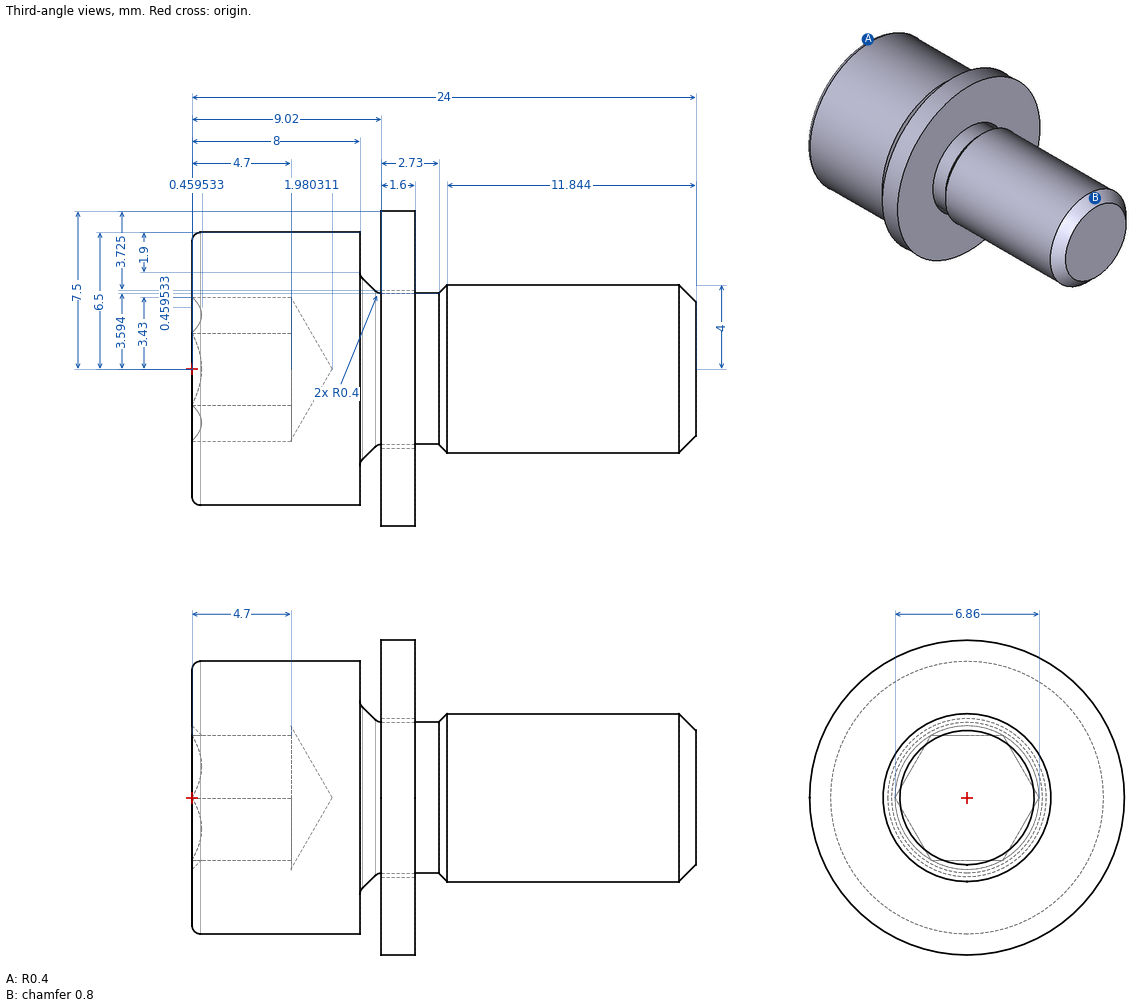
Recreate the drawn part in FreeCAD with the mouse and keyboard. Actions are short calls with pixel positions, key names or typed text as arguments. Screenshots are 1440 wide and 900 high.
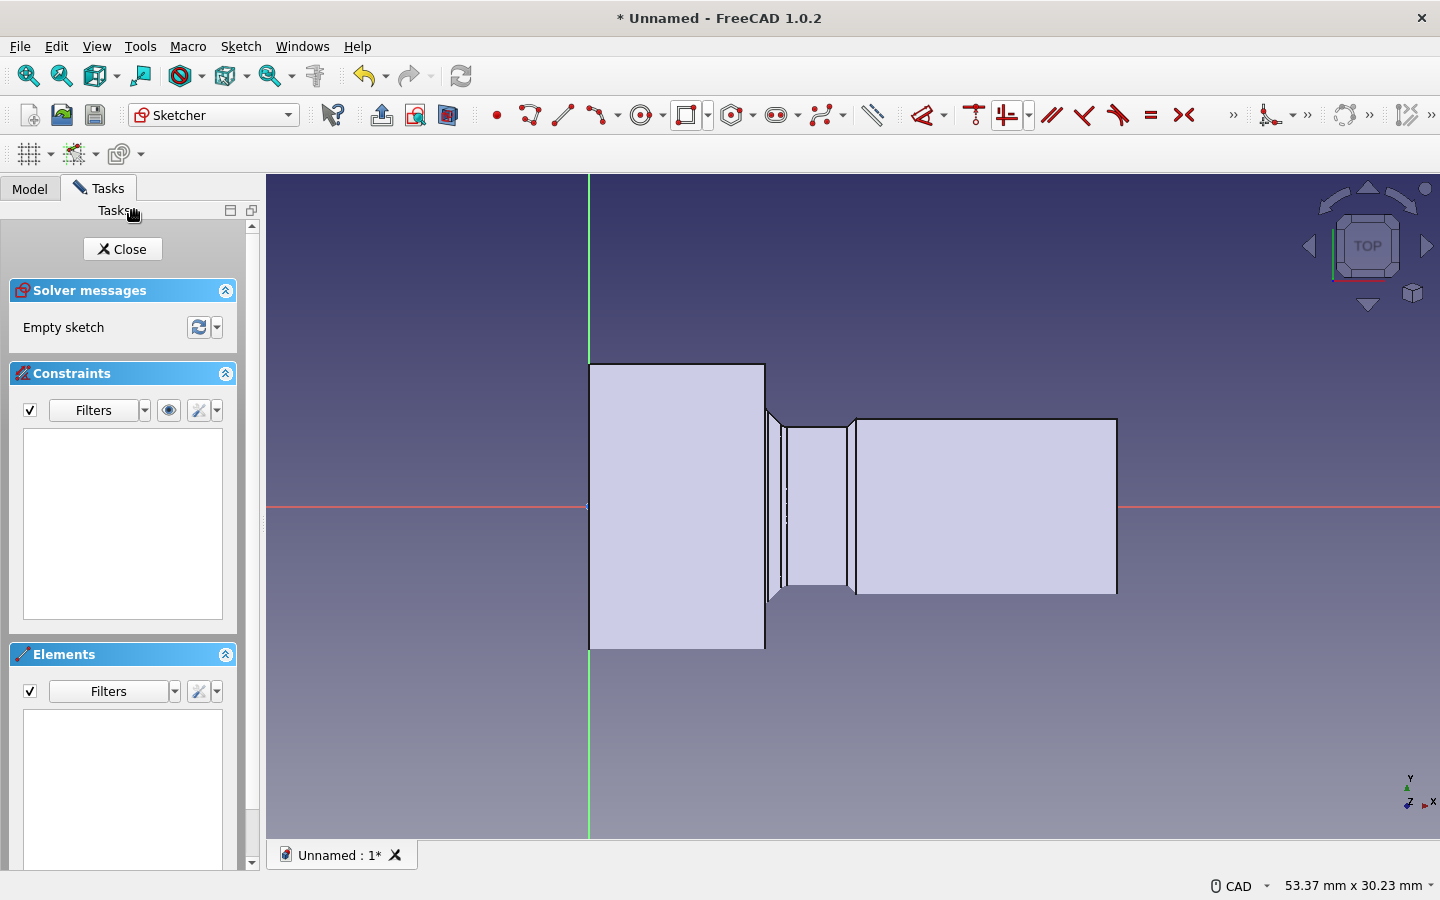
click(448, 116)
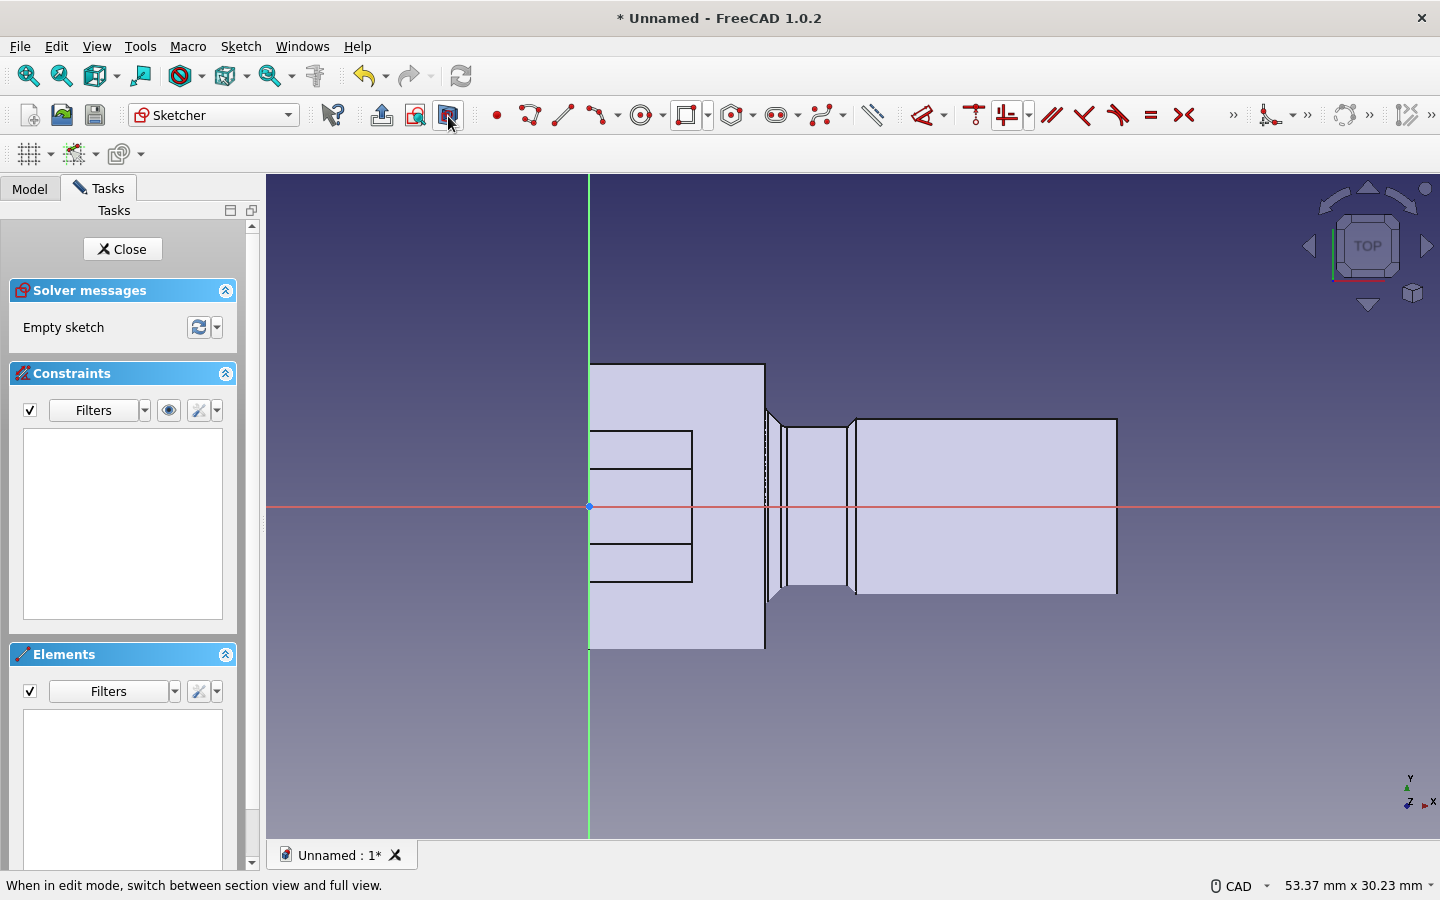
scroll(584, 432, up, 15)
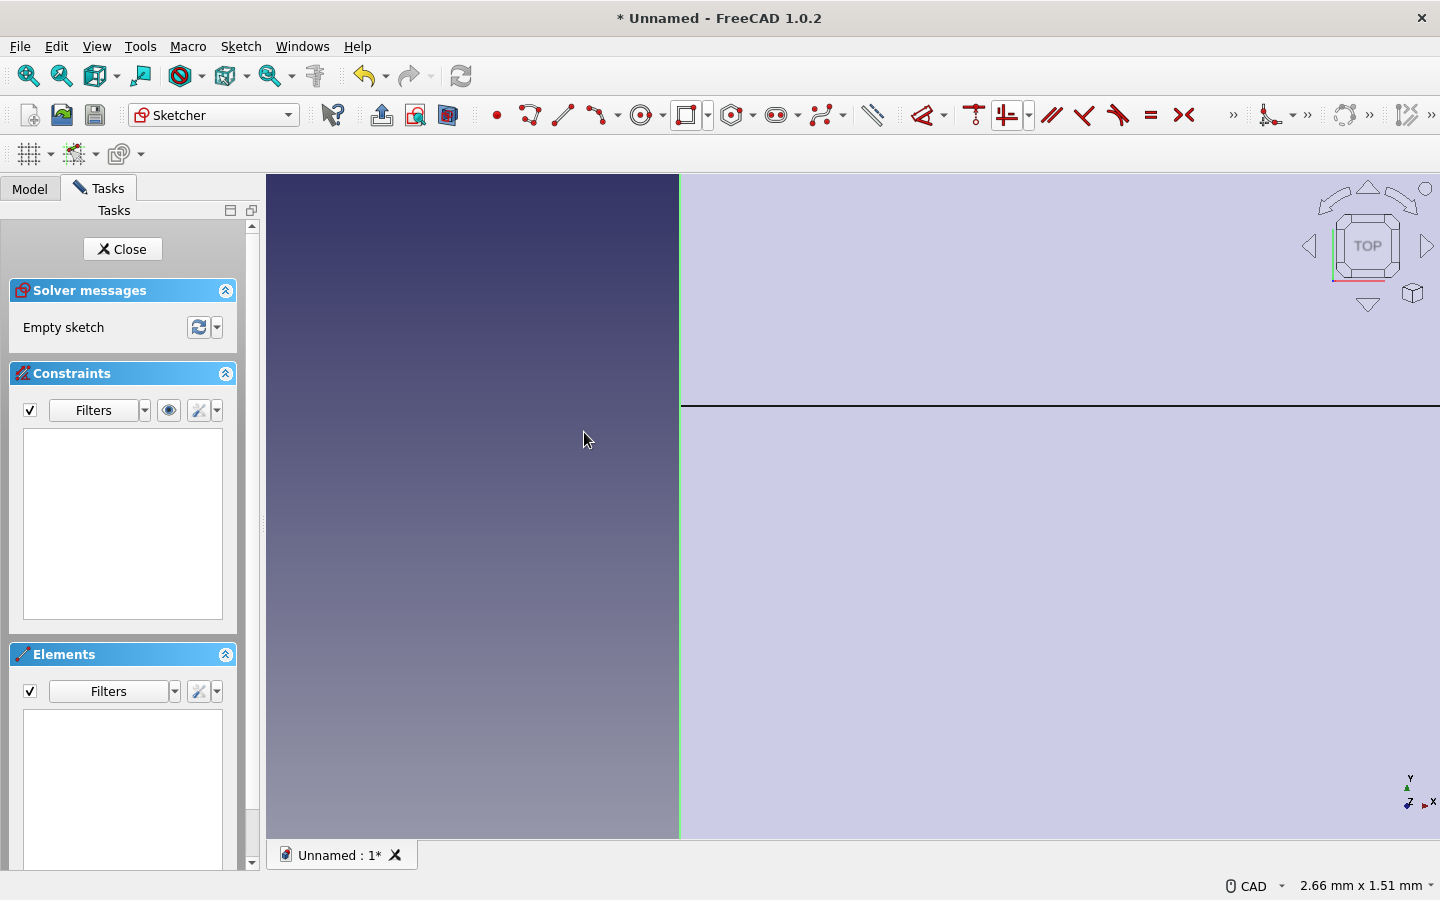
scroll(779, 508, up, 4)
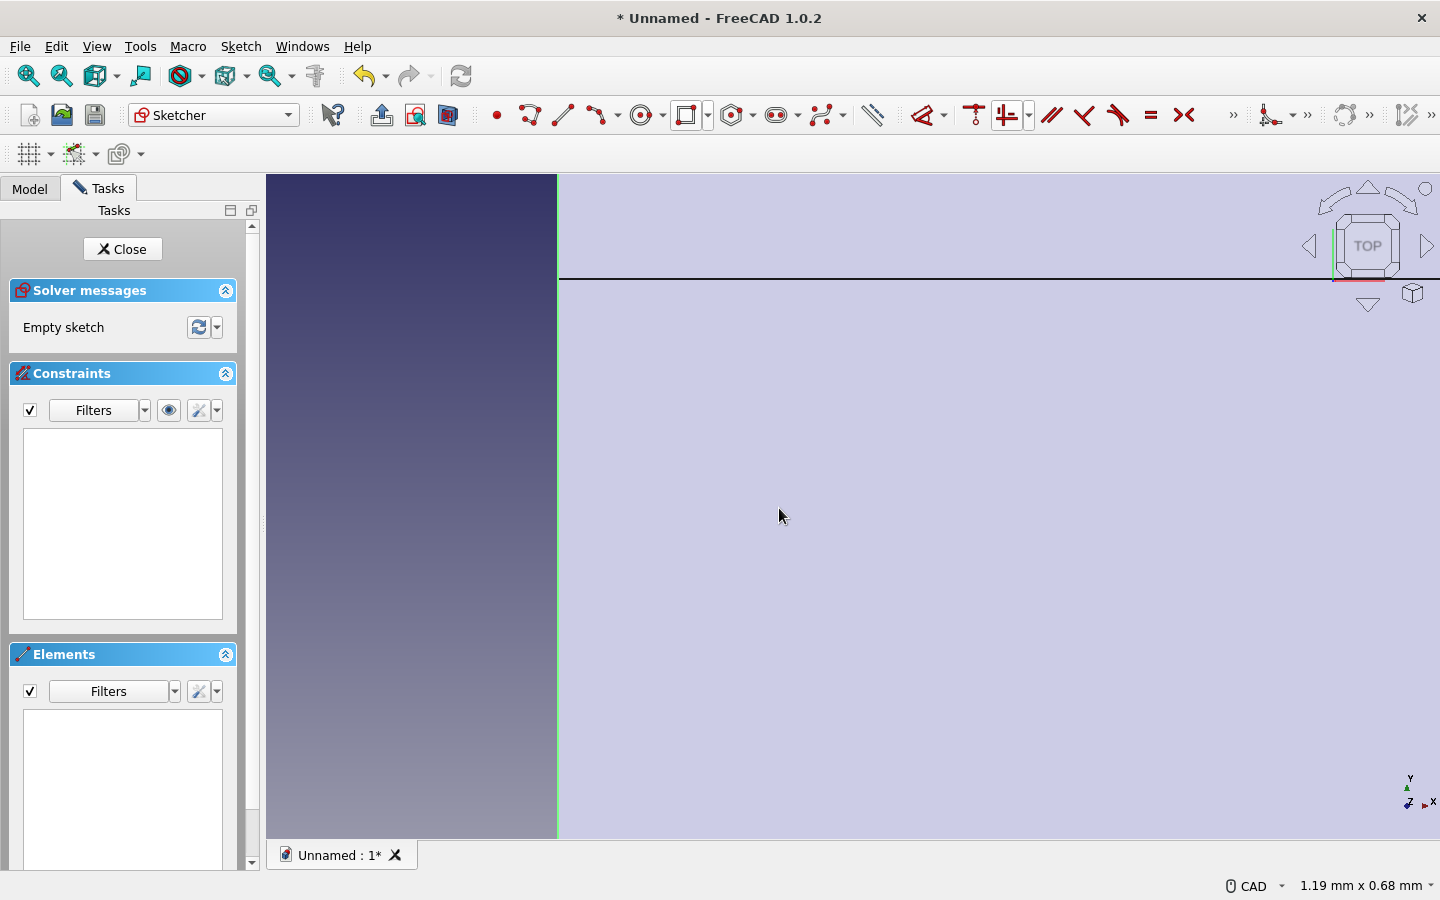
click(530, 116)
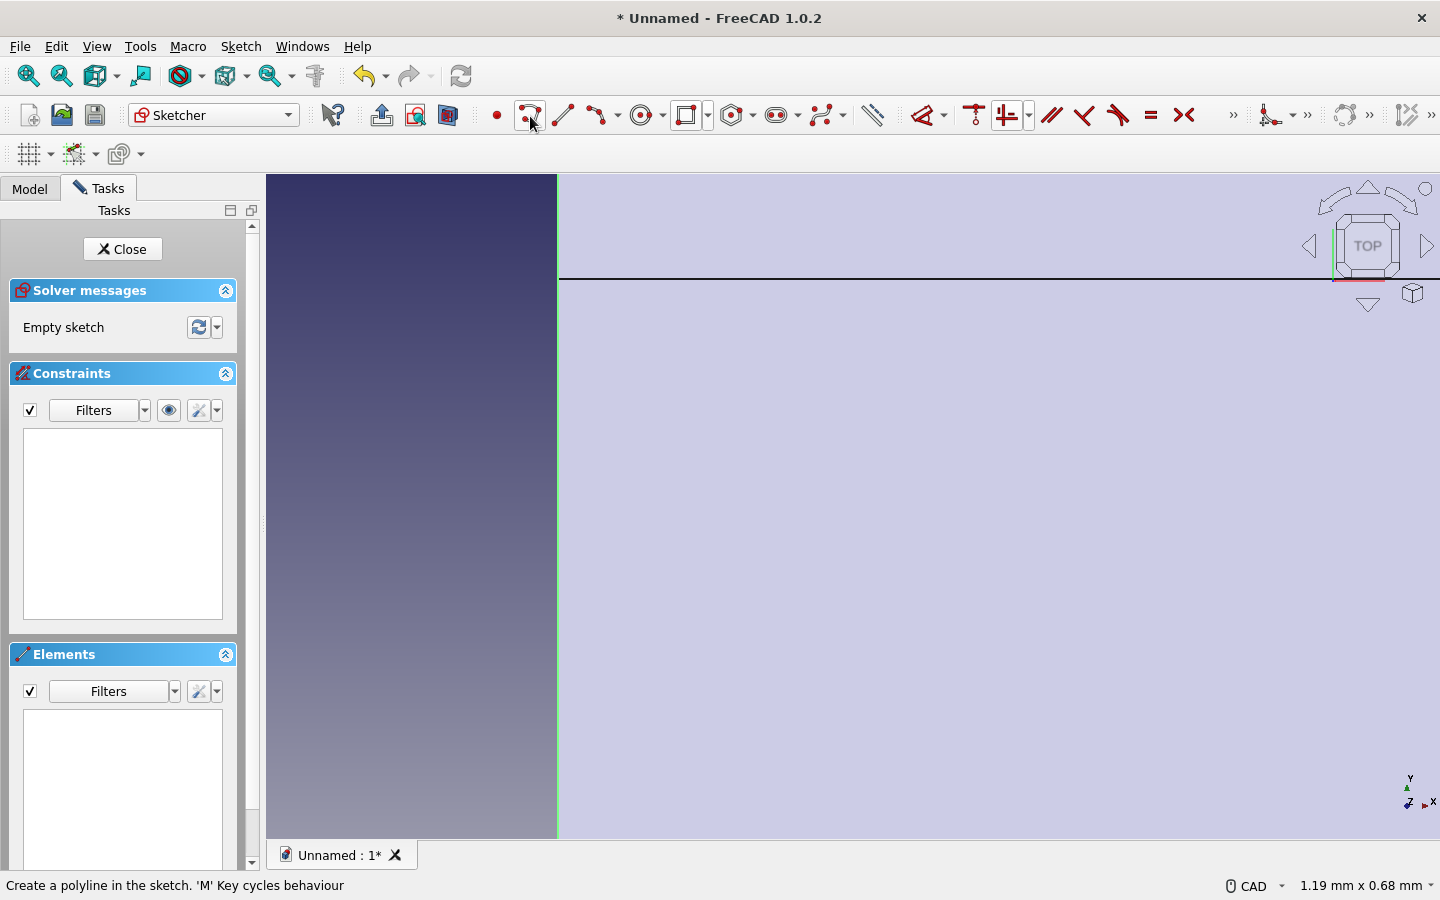
click(558, 731)
click(1010, 731)
click(567, 279)
click(558, 732)
key(Escape)
key(Escape)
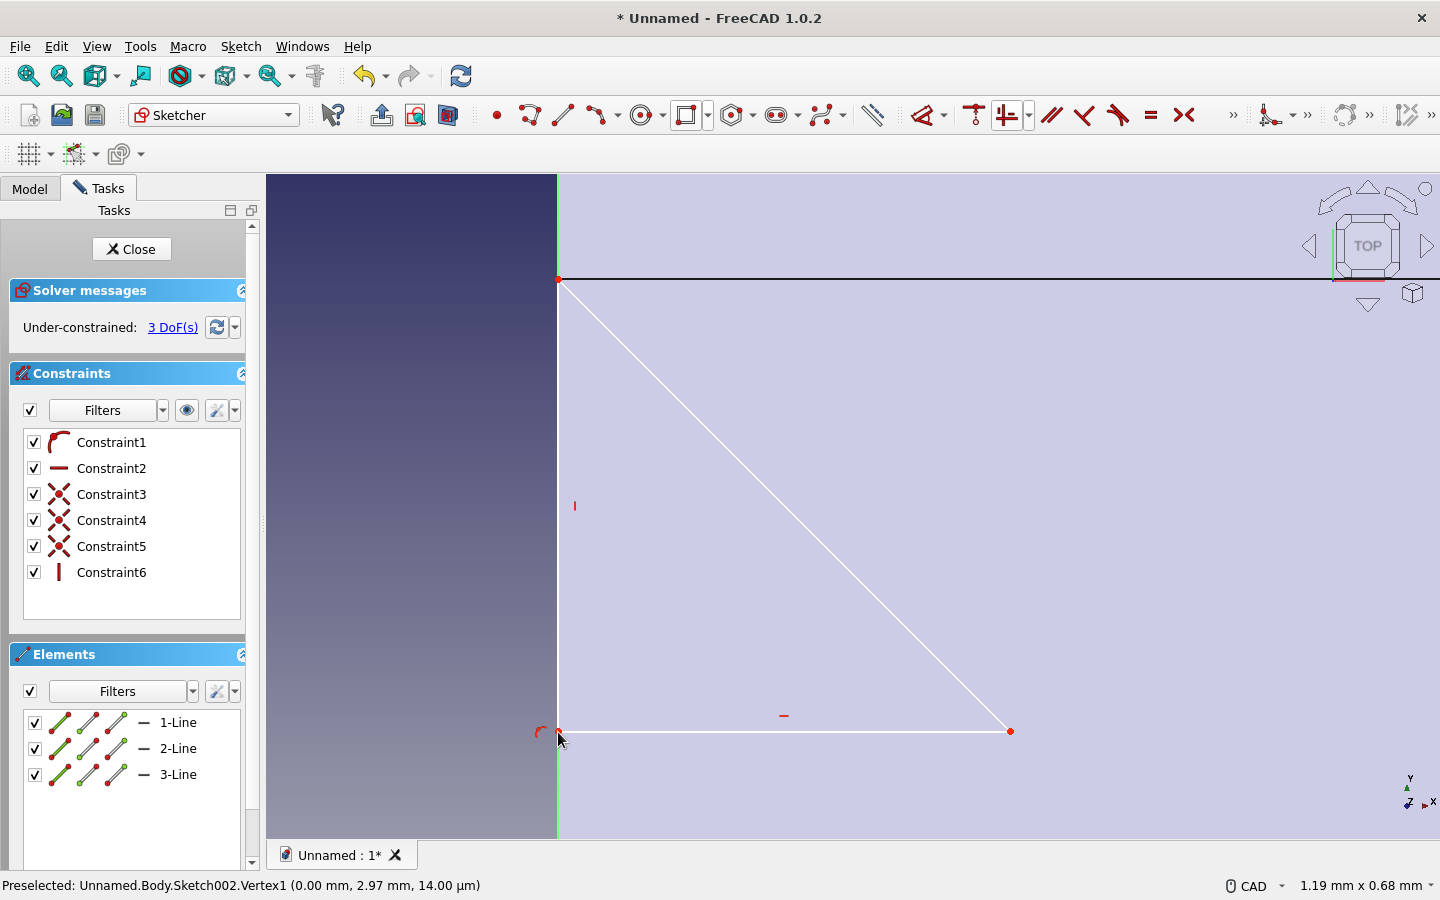
click(922, 116)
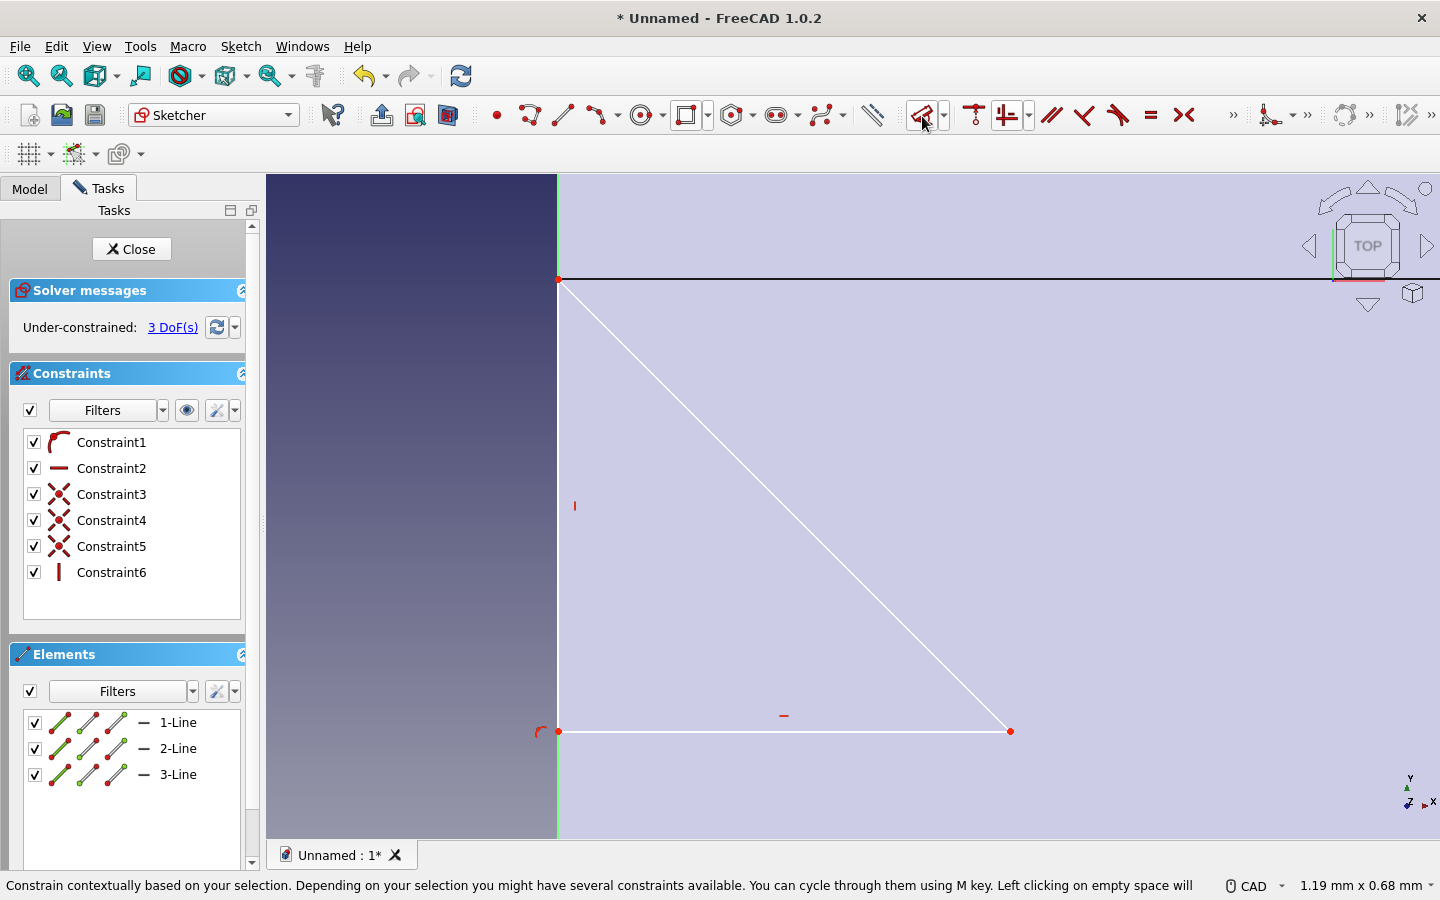
click(558, 280)
click(524, 545)